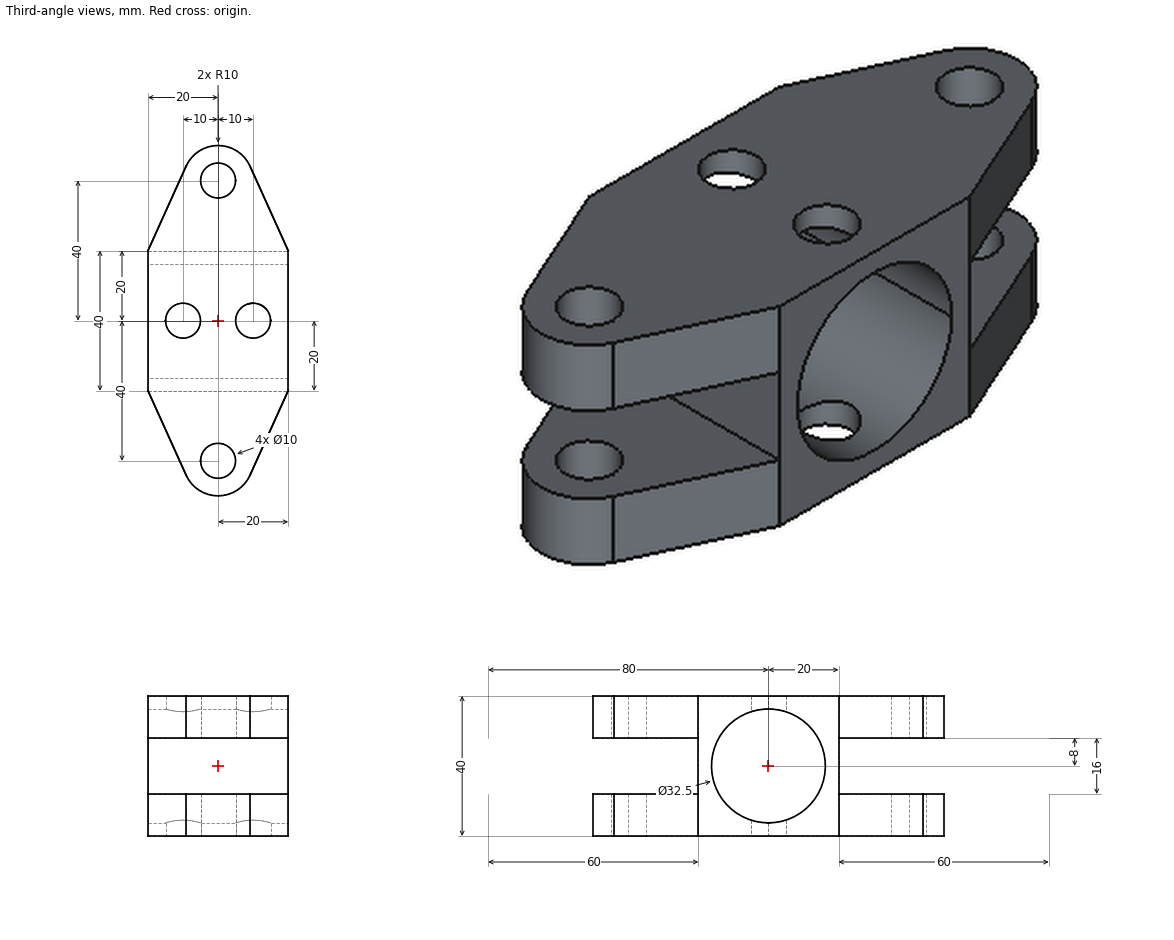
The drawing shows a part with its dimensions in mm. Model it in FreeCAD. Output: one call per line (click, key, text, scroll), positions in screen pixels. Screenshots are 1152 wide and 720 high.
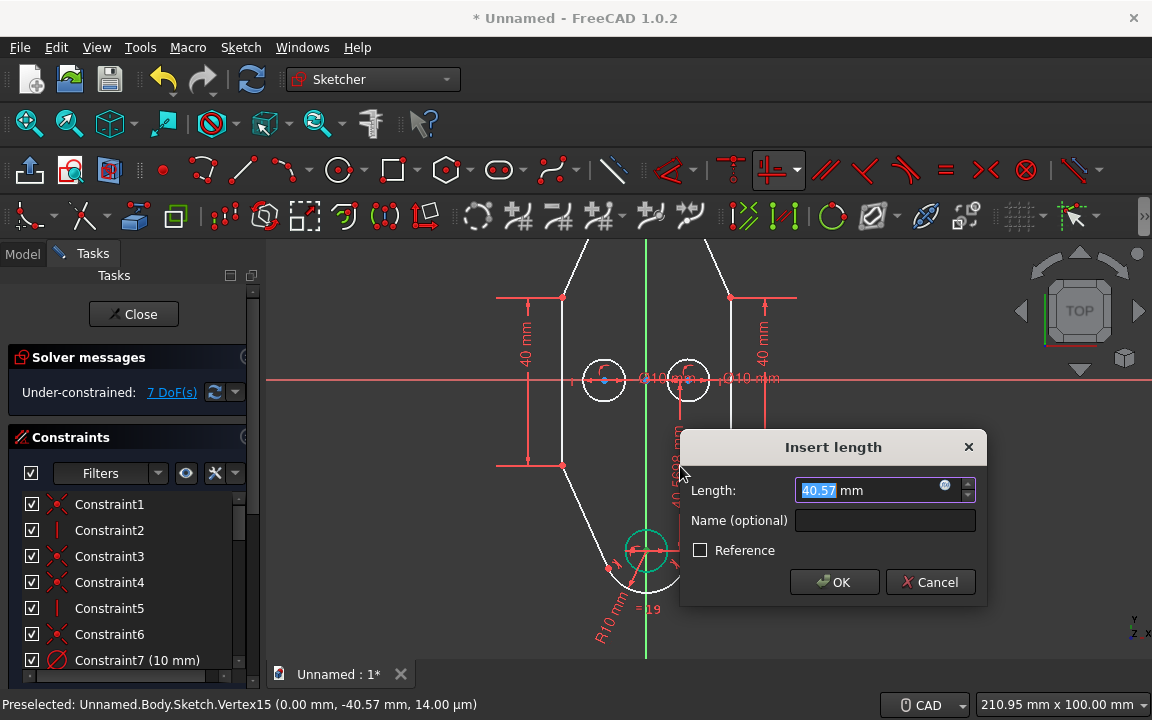
text(40)
key(Return)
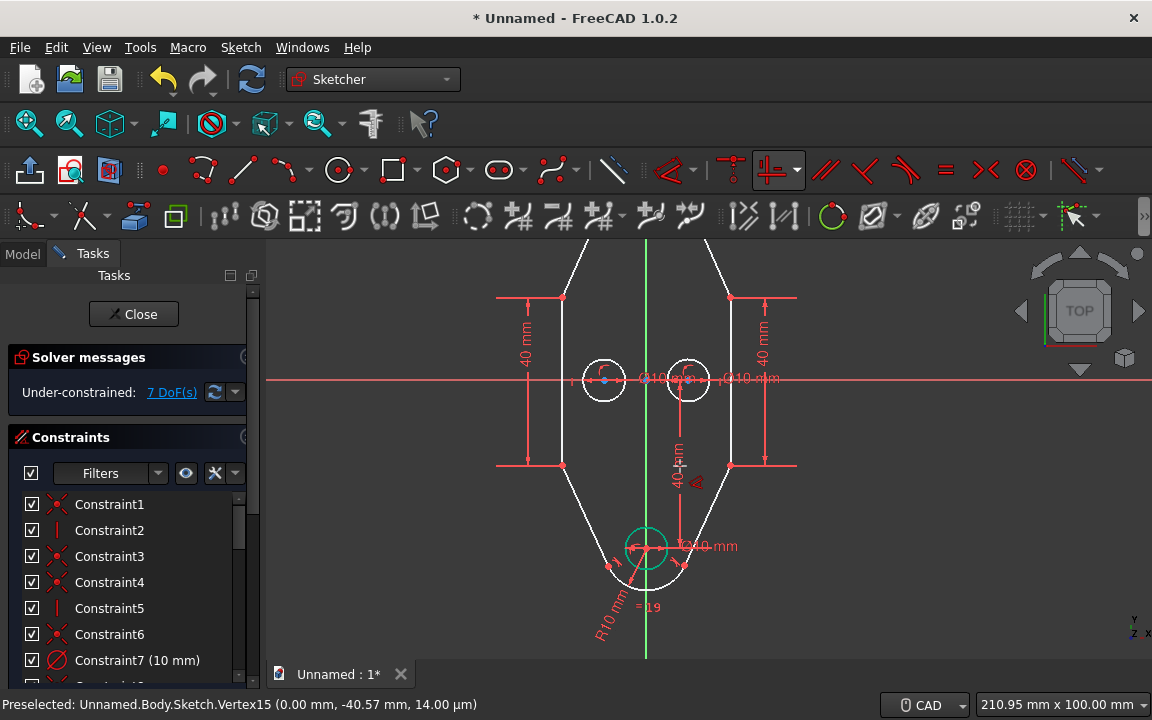
click(604, 380)
click(625, 414)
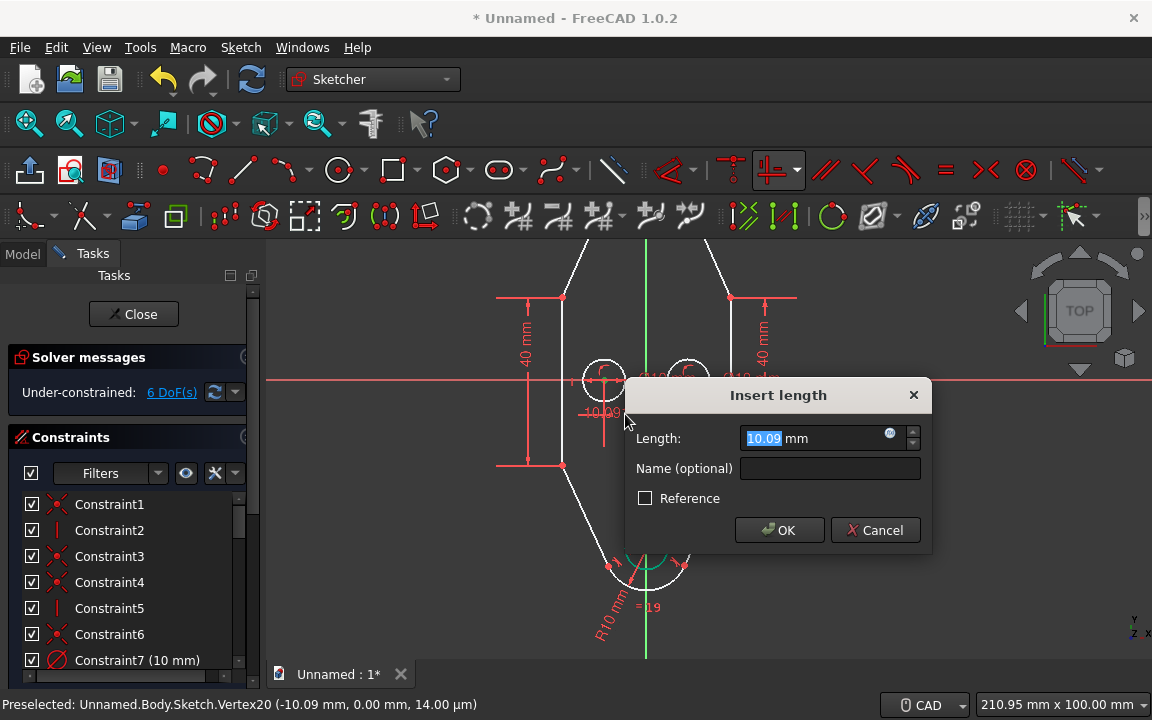
text(10)
key(Return)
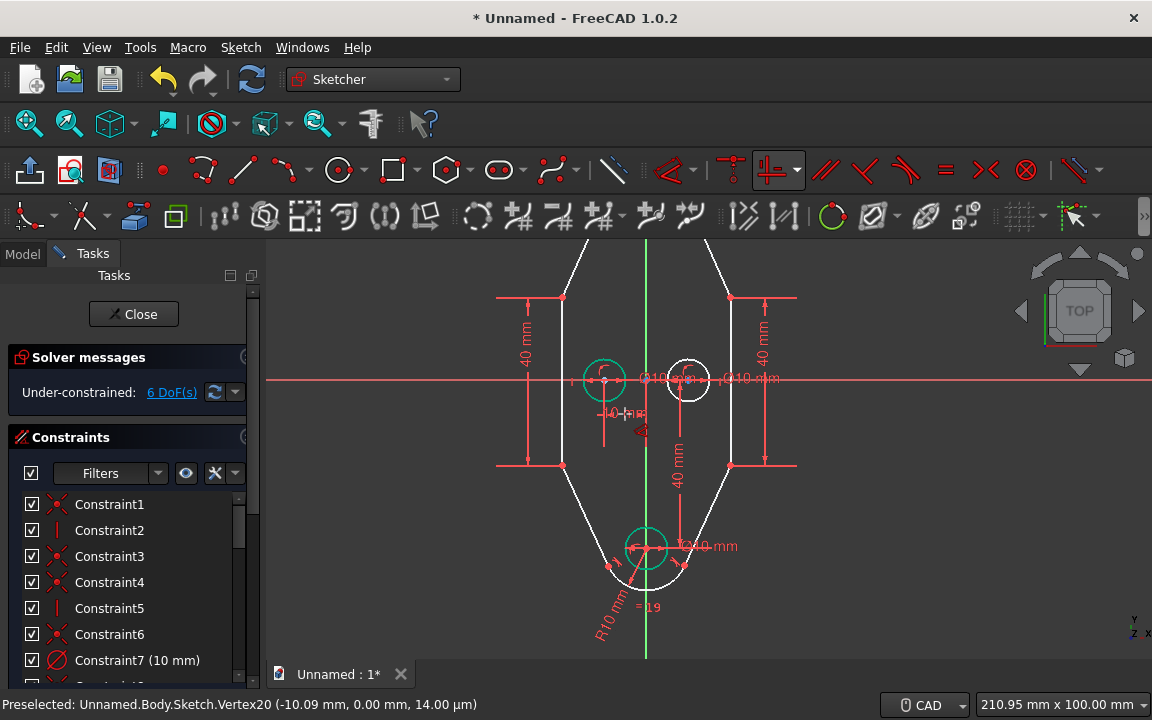
click(688, 380)
click(667, 346)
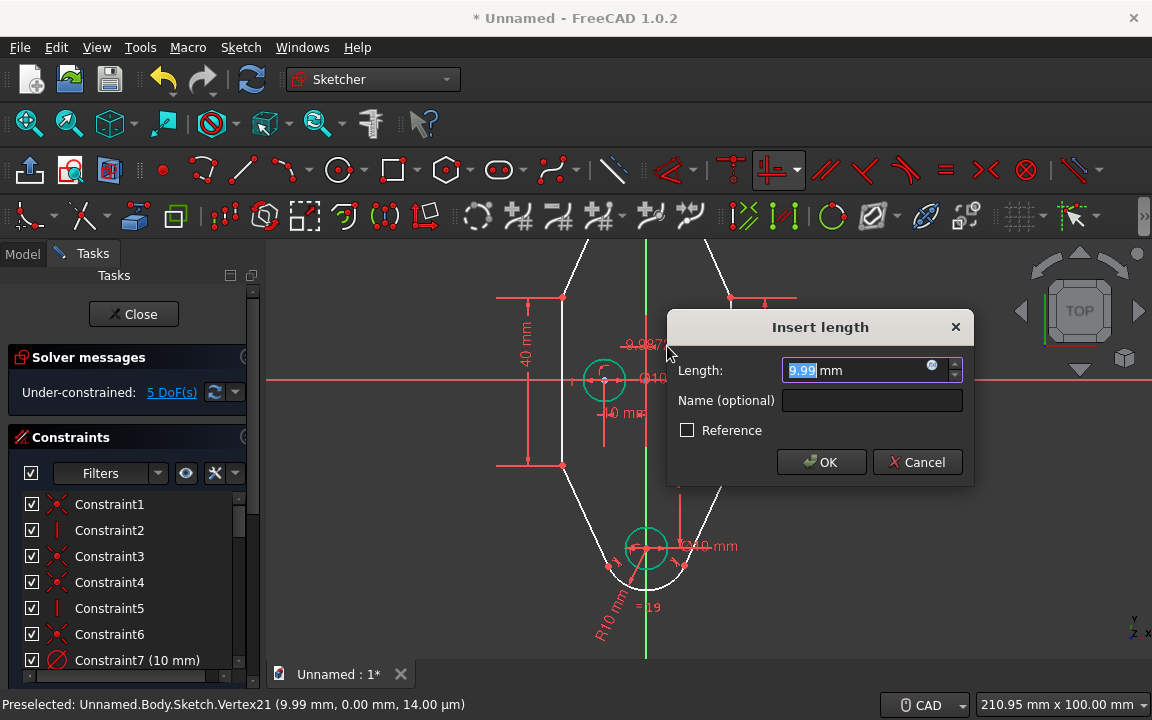
text(10)
key(Return)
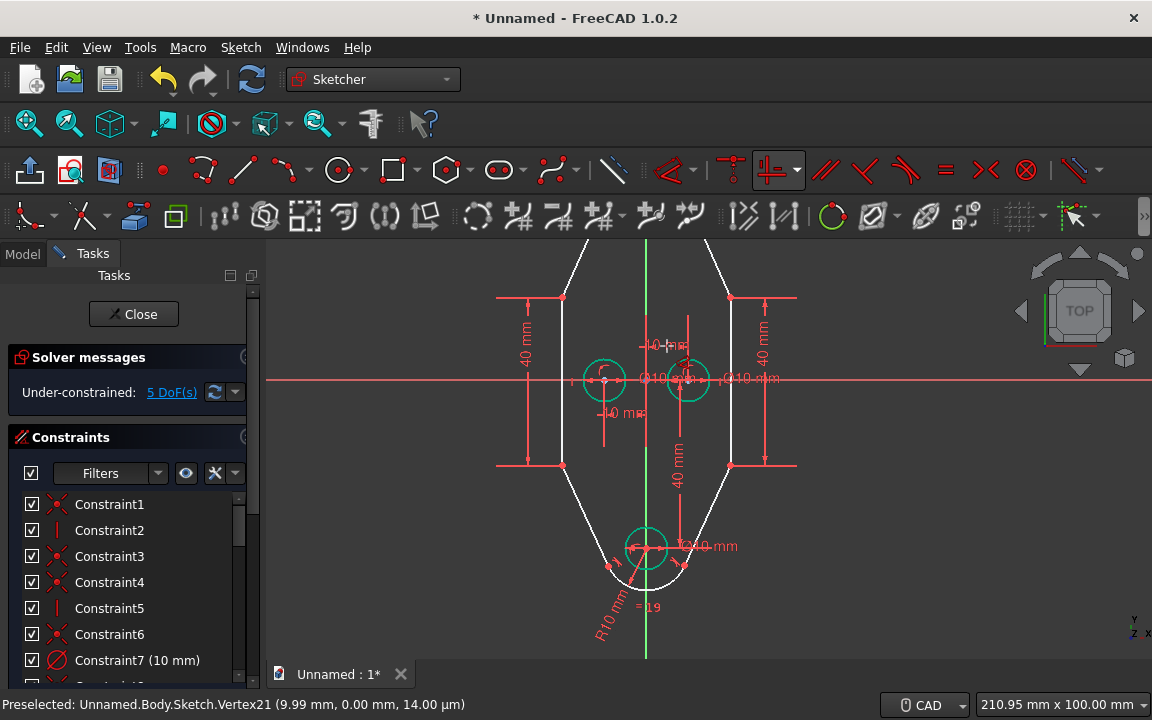
scroll(628, 588, down, 2)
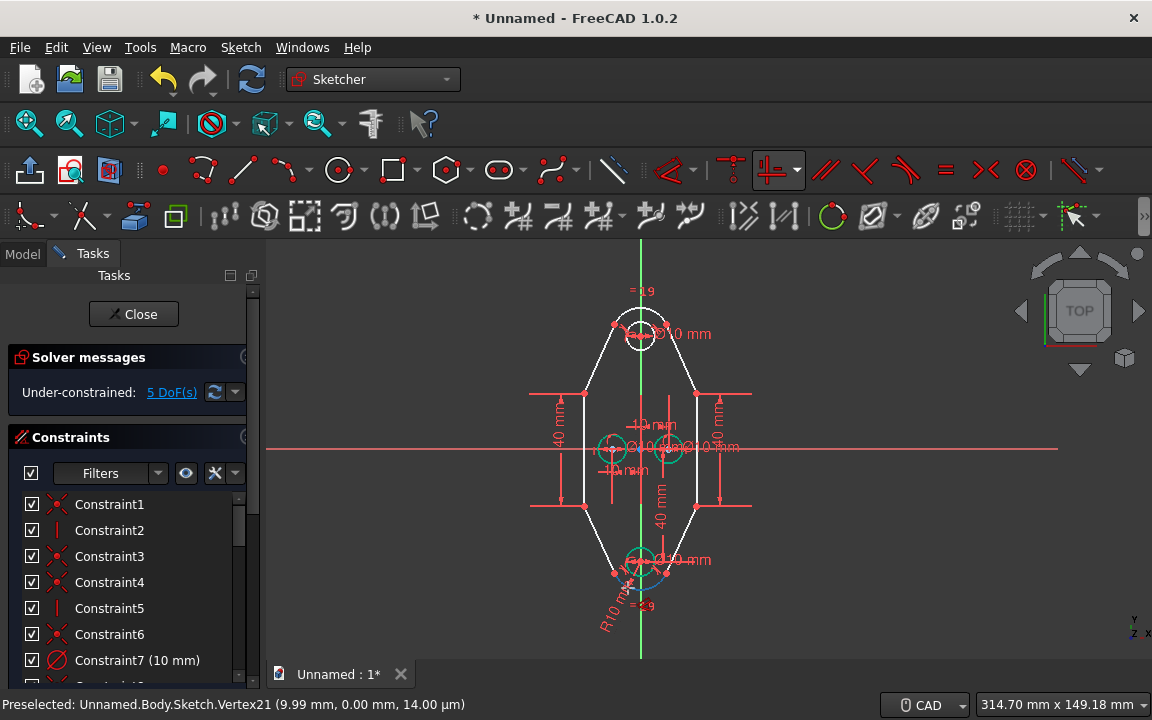
click(641, 336)
click(675, 393)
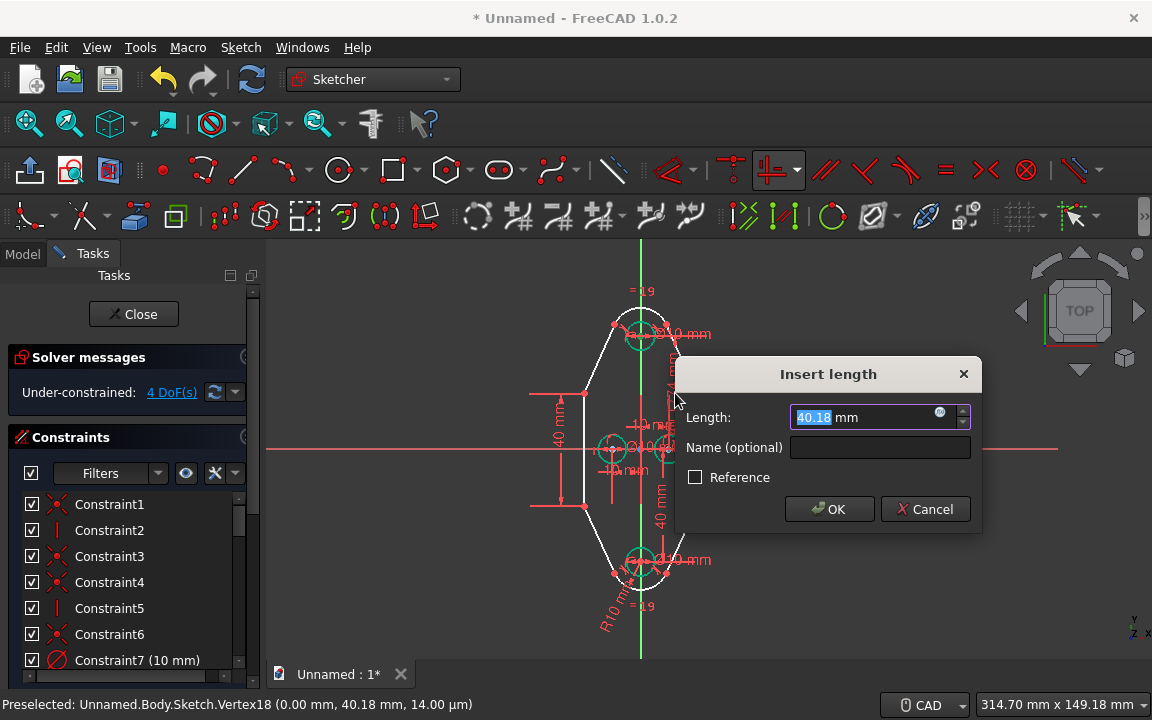
text(40)
key(Return)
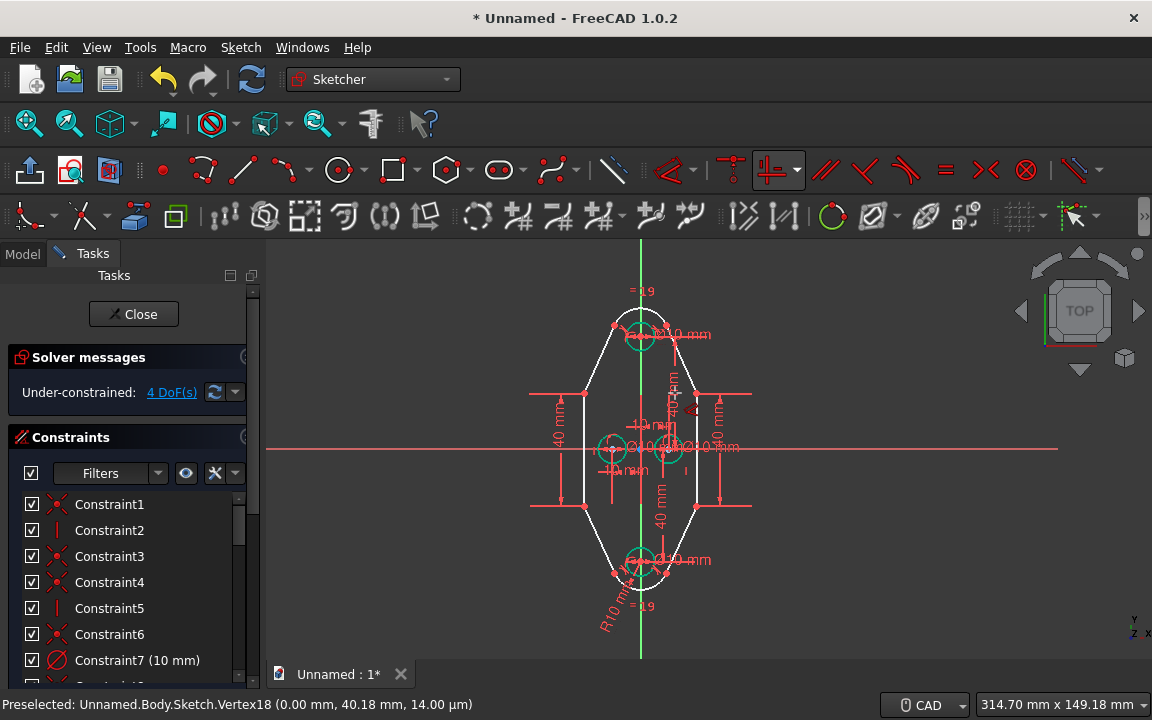
click(584, 394)
click(625, 360)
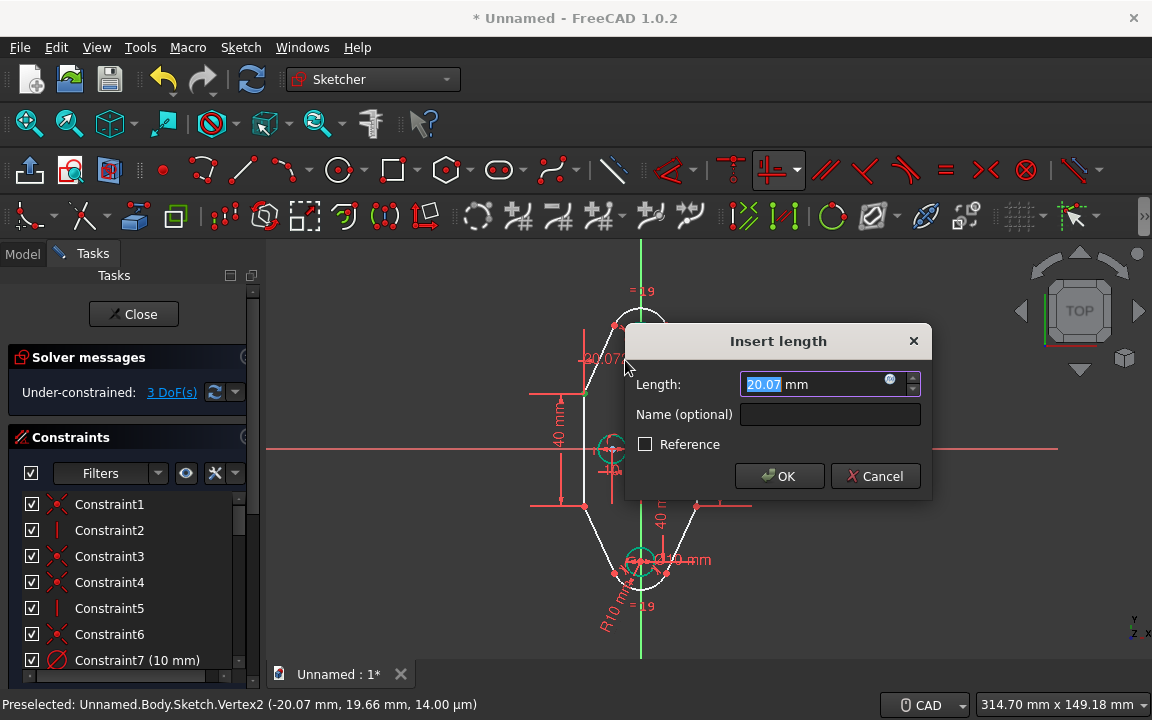
text(20)
key(Return)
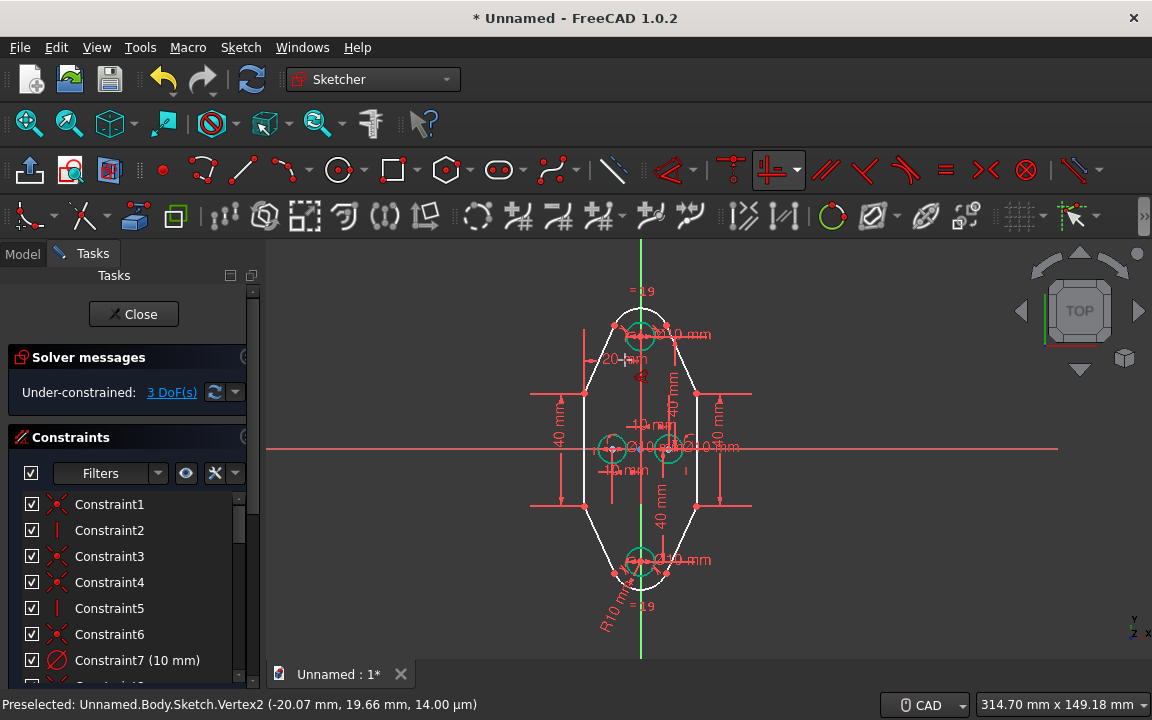
click(584, 394)
click(550, 402)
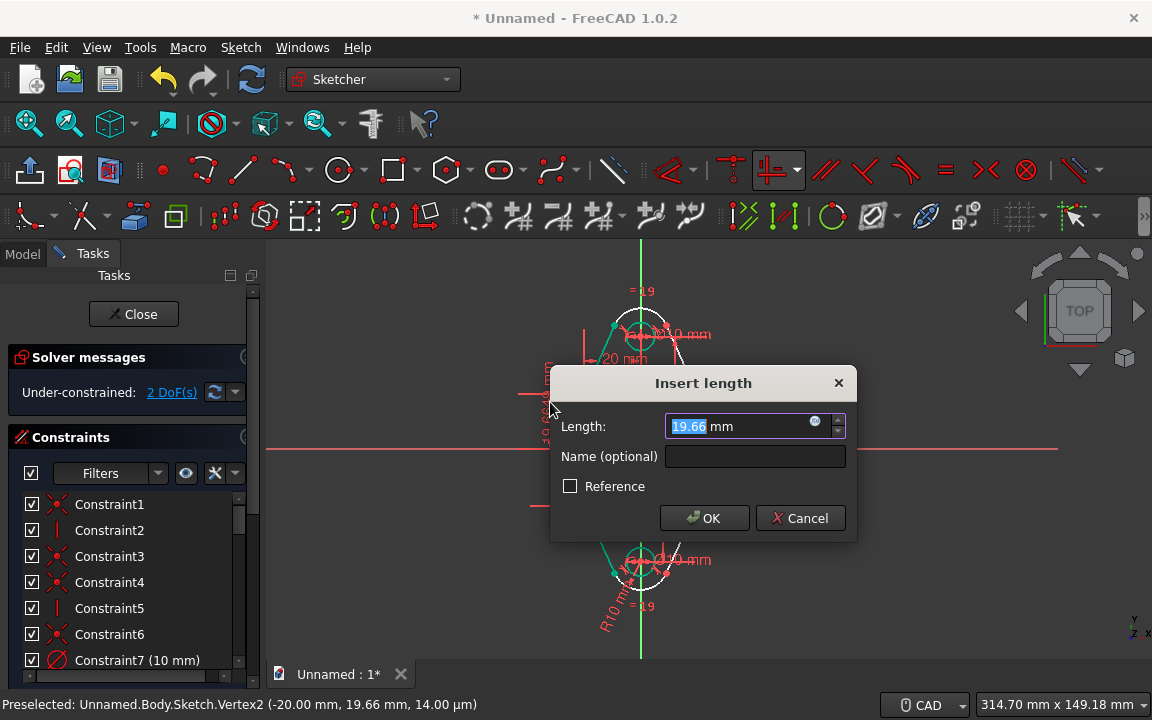
text(20)
key(Return)